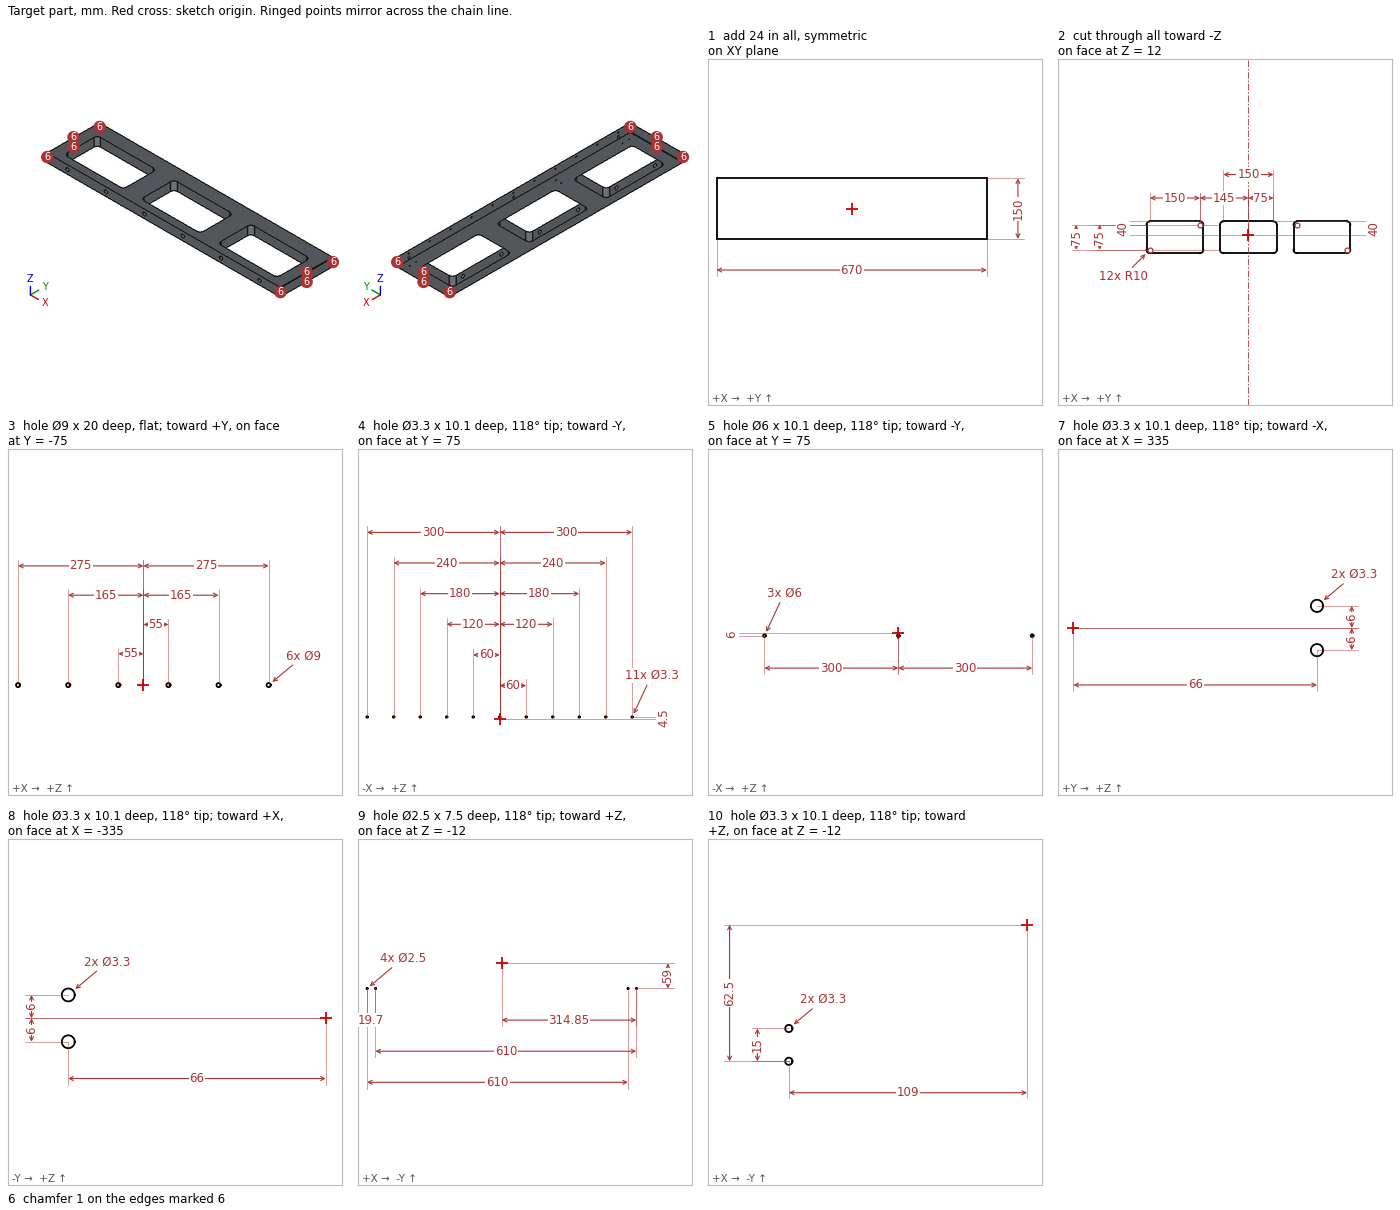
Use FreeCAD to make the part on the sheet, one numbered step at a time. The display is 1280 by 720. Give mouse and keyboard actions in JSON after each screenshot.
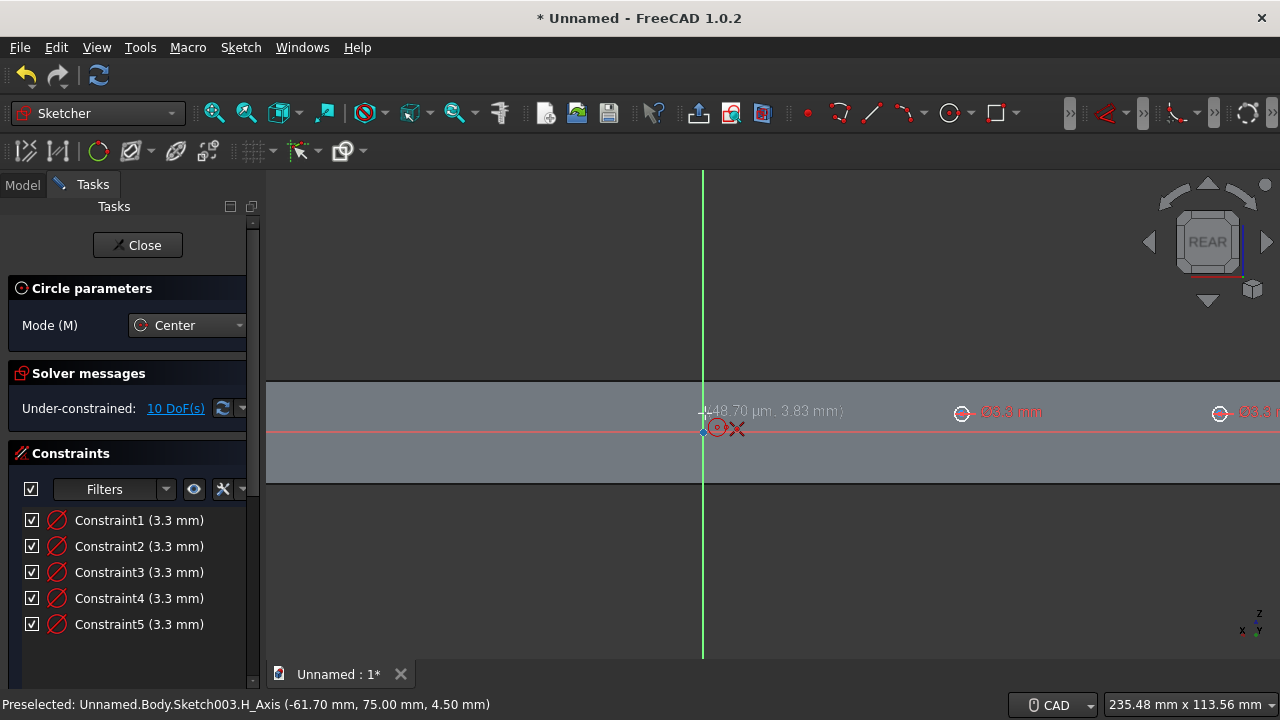
{"action": "left_click", "coordinate": [703, 413]}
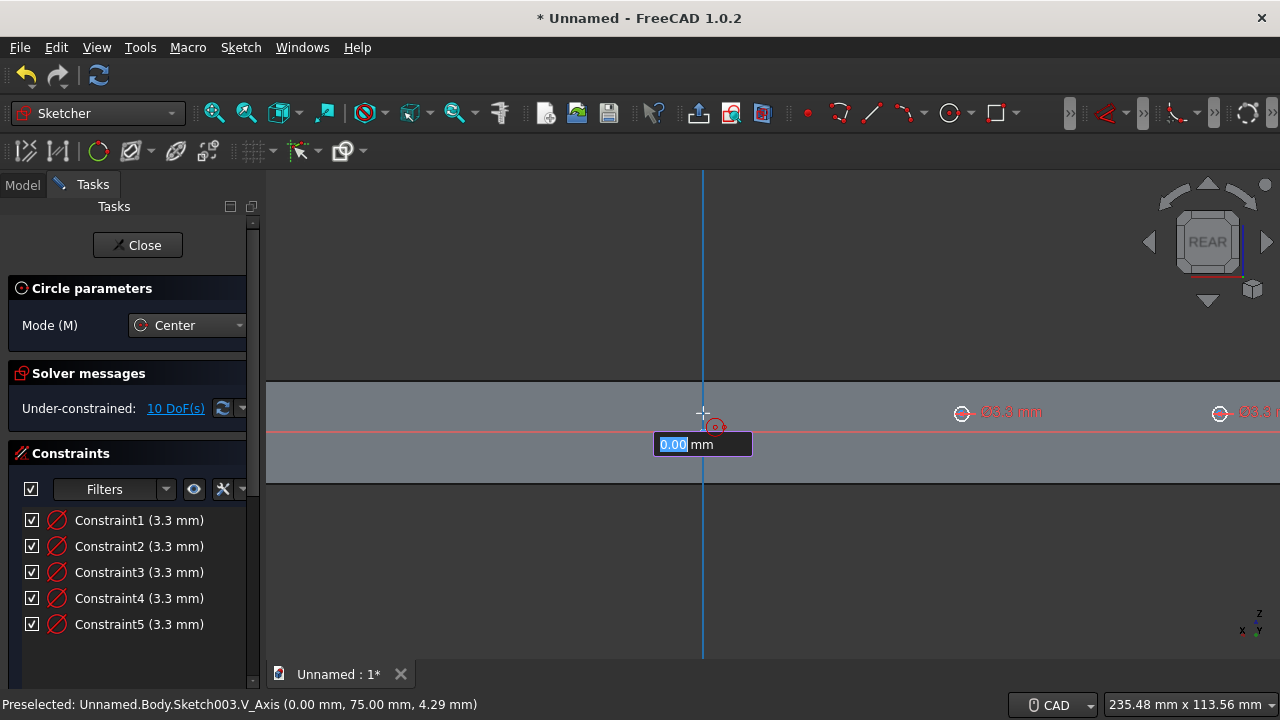
{"action": "scroll", "coordinate": [710, 411], "scroll_direction": "up", "scroll_amount": 5}
{"action": "mouse_move", "coordinate": [709, 409]}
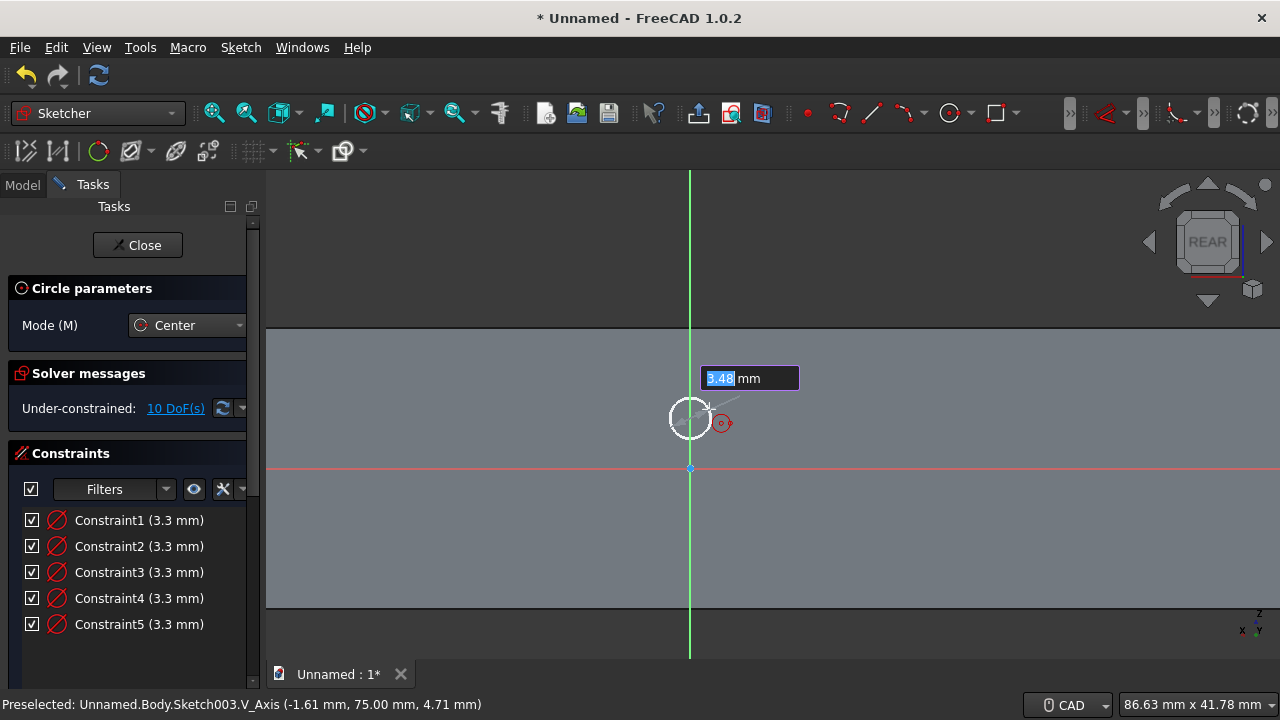
{"action": "type", "text": "3.3"}
{"action": "key", "text": "Return"}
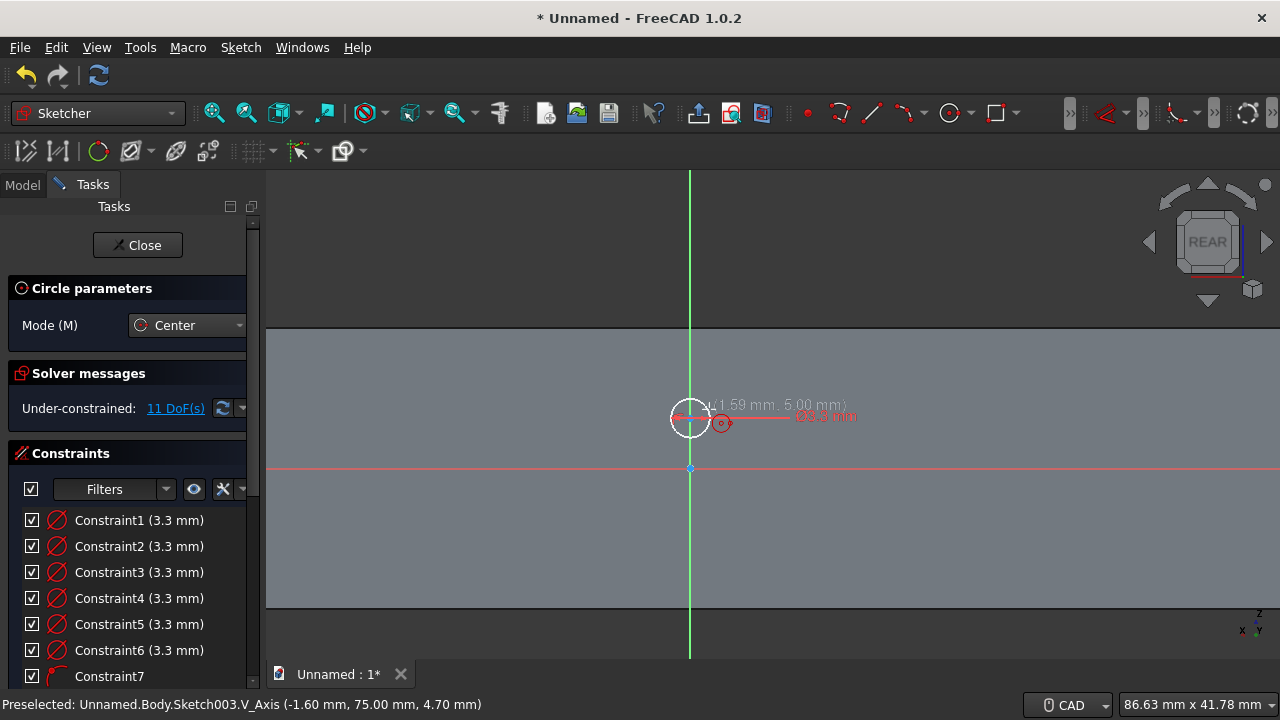
{"action": "scroll", "coordinate": [706, 413], "scroll_direction": "down", "scroll_amount": 13}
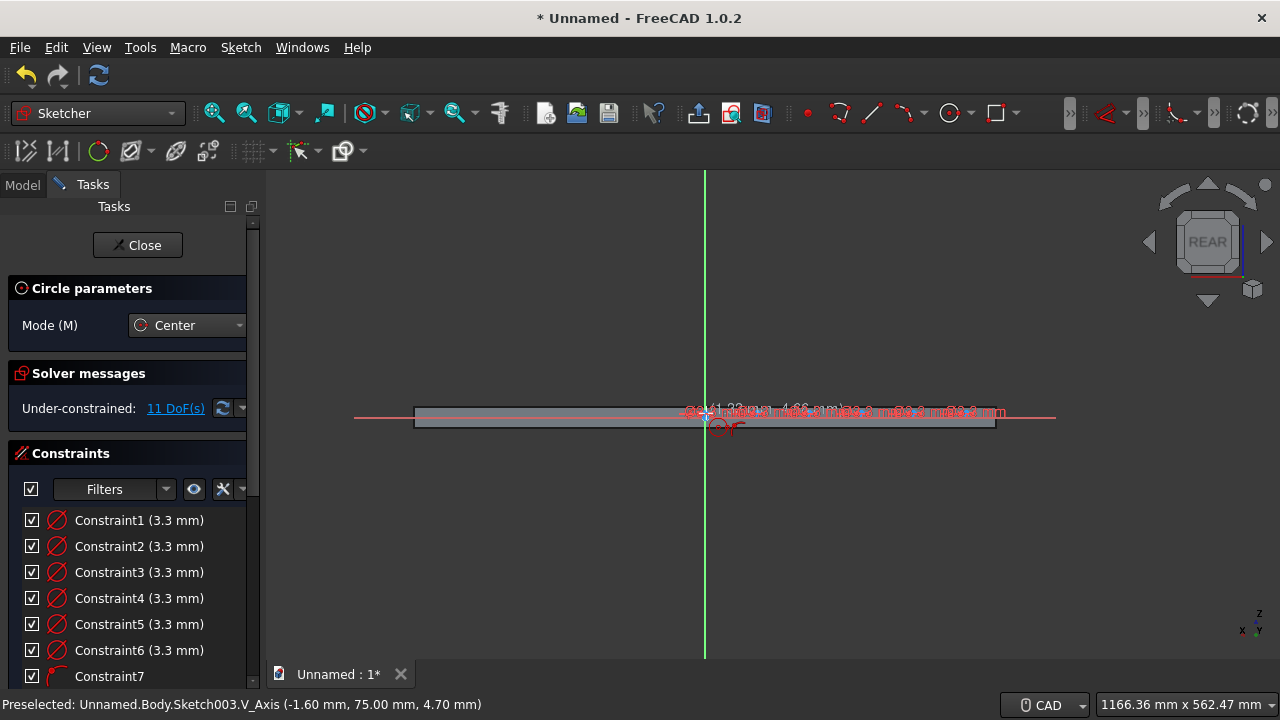
{"action": "scroll", "coordinate": [653, 414], "scroll_direction": "up", "scroll_amount": 14}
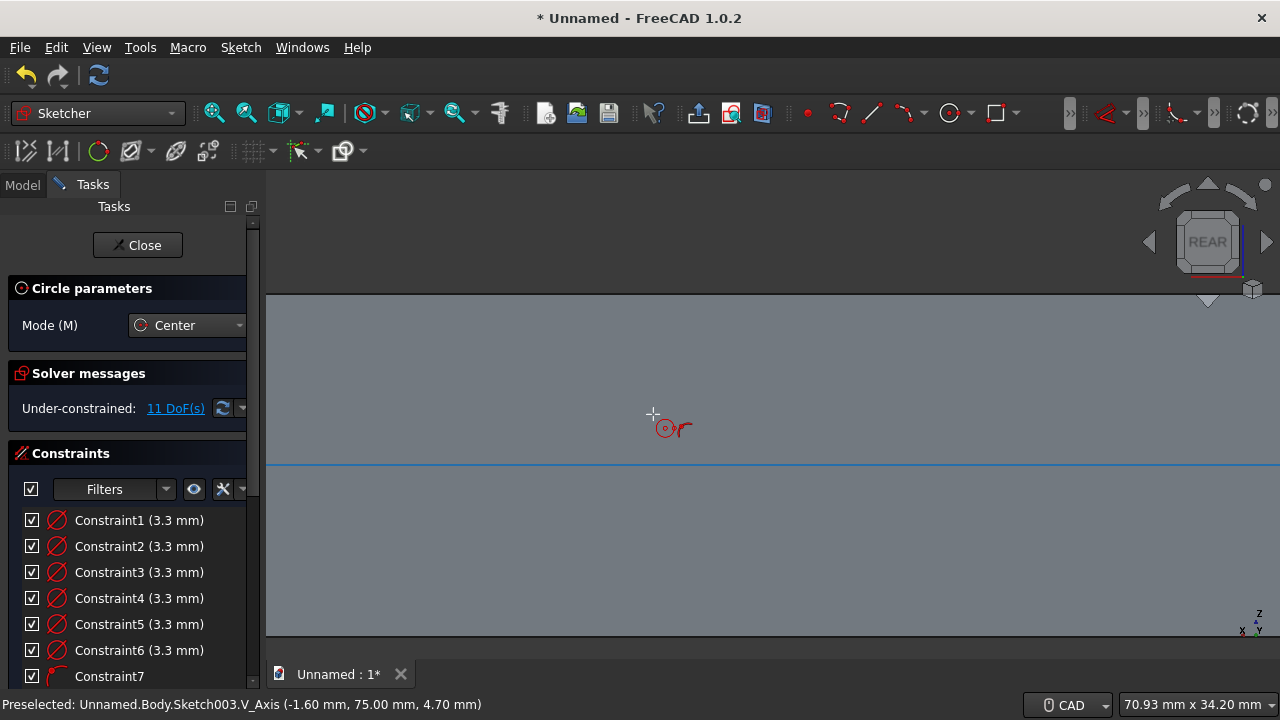
{"action": "scroll", "coordinate": [653, 414], "scroll_direction": "down", "scroll_amount": 14}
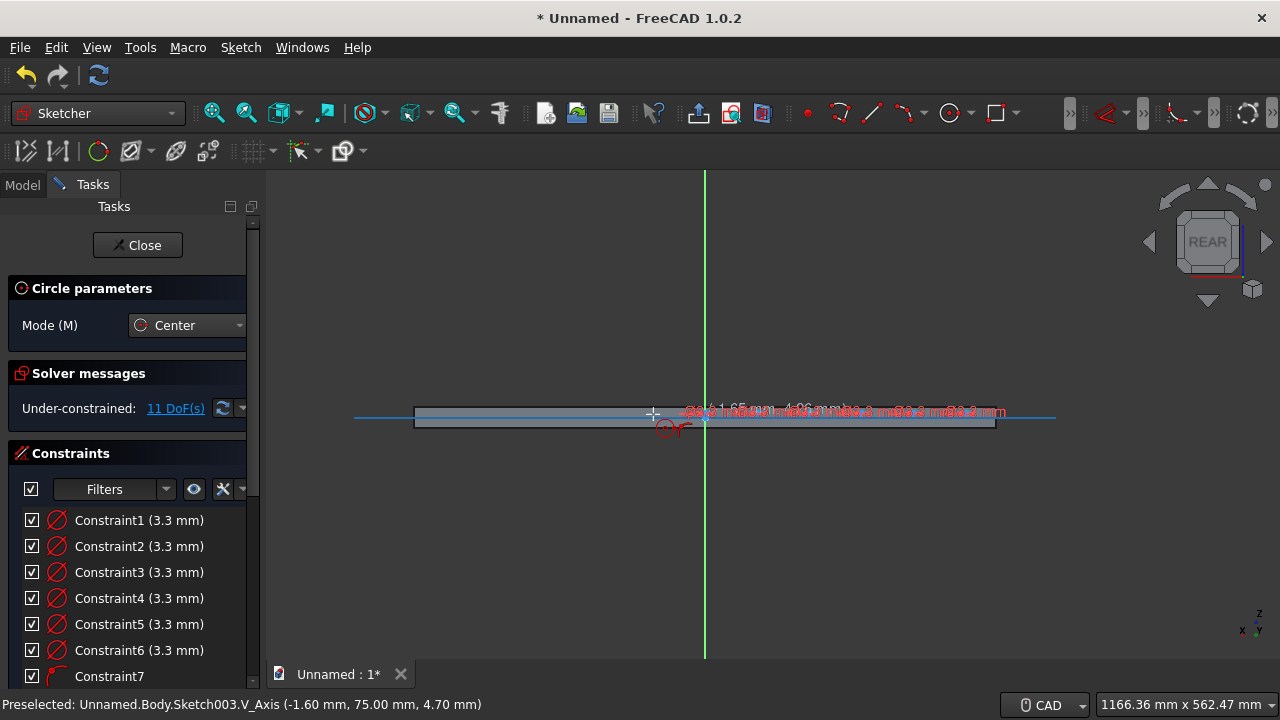
{"action": "scroll", "coordinate": [653, 414], "scroll_direction": "up", "scroll_amount": 8}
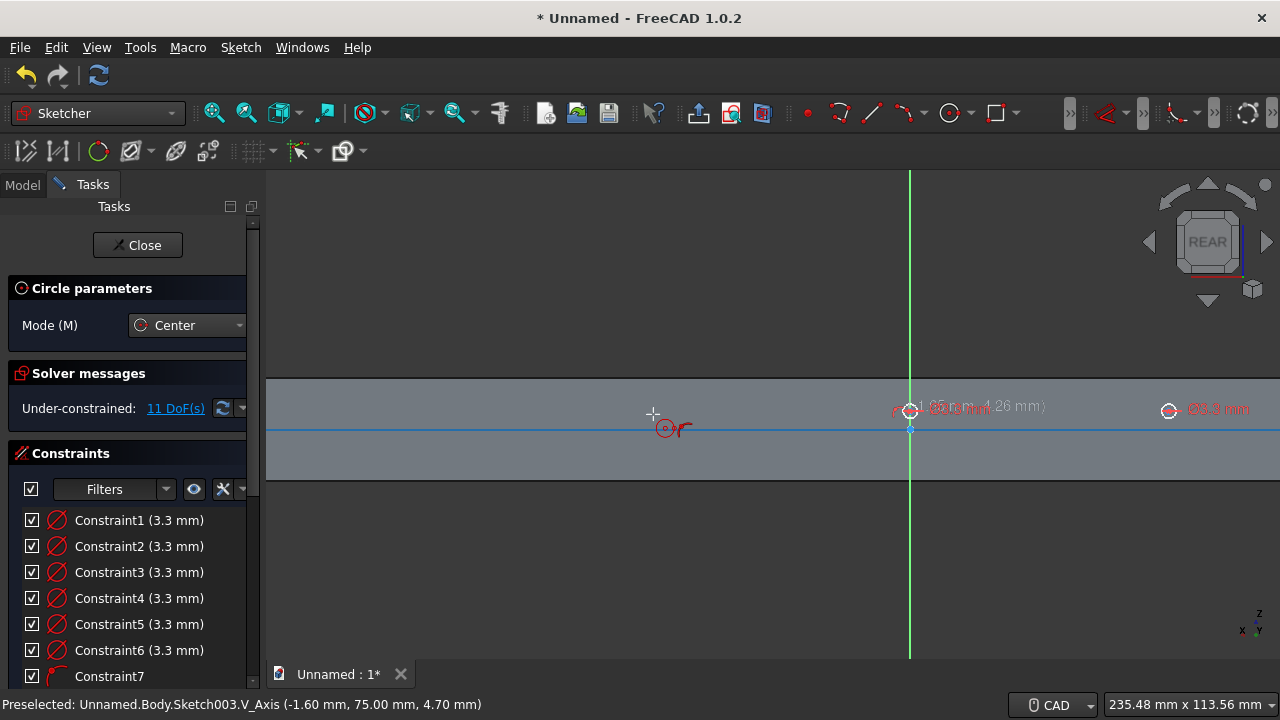
{"action": "left_click", "coordinate": [652, 410]}
{"action": "mouse_move", "coordinate": [657, 405]}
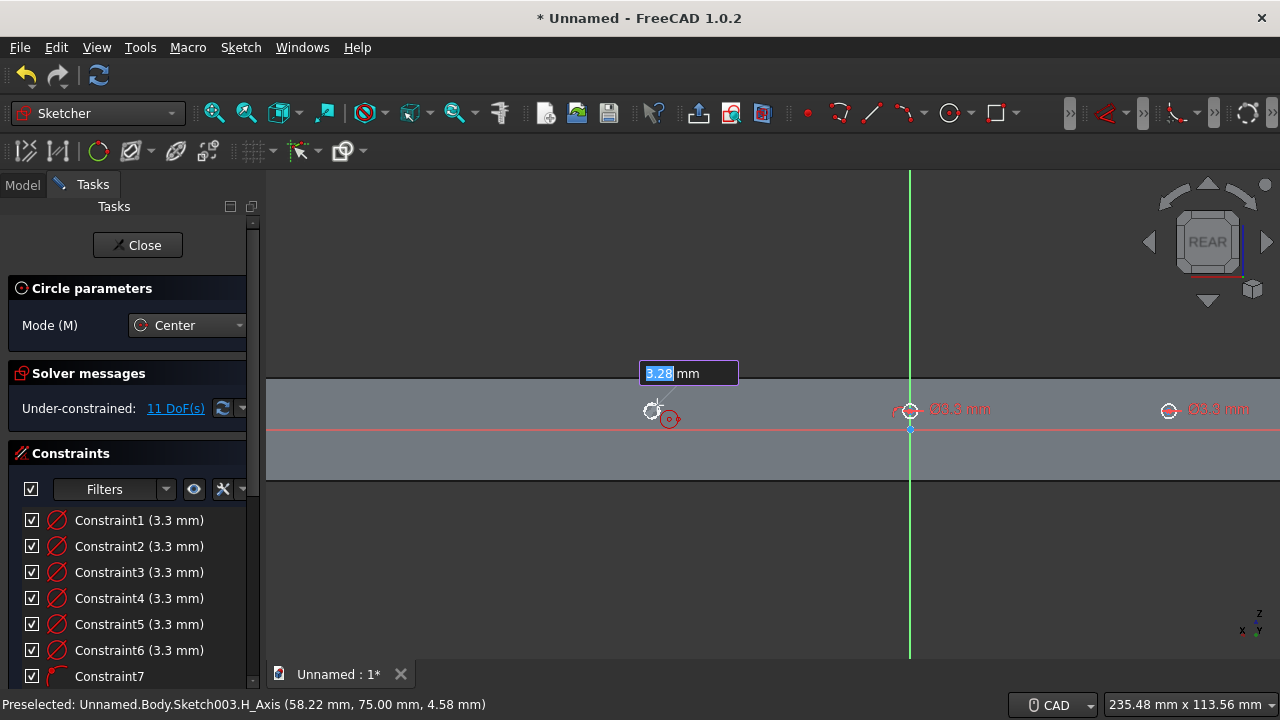
{"action": "type", "text": "3.3"}
{"action": "key", "text": "Return"}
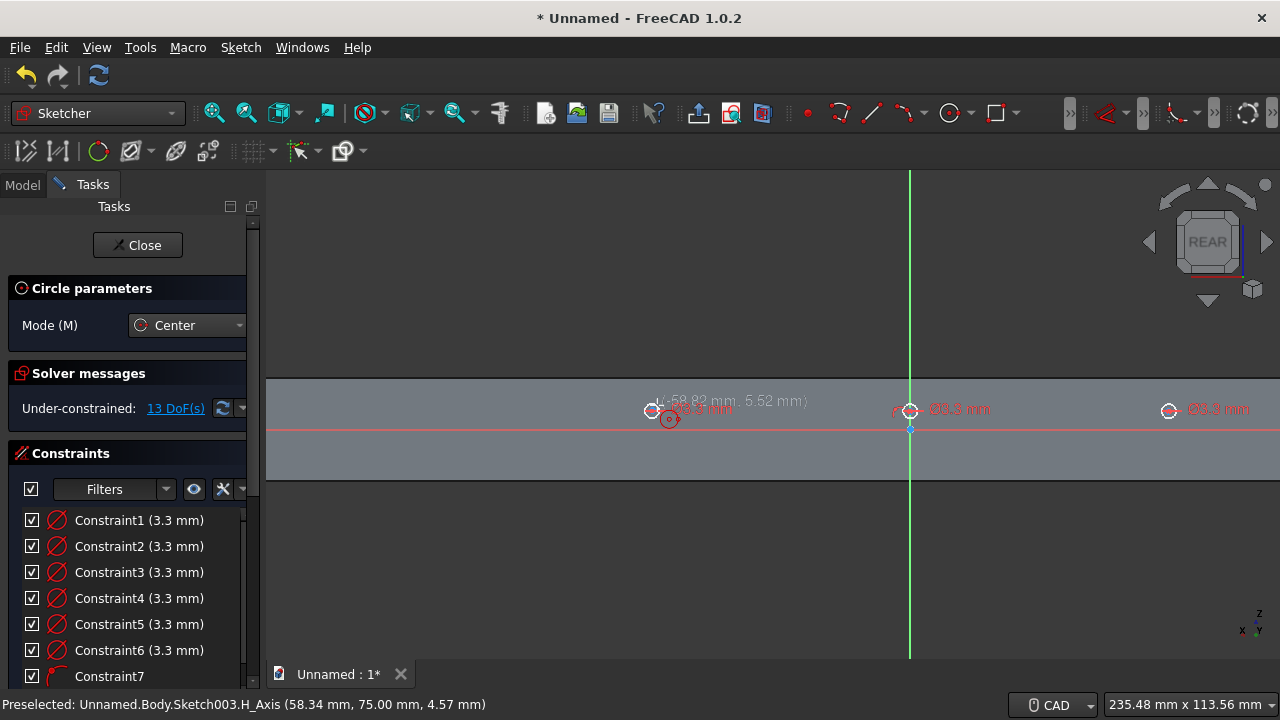
{"action": "scroll", "coordinate": [394, 410], "scroll_direction": "up", "scroll_amount": 6}